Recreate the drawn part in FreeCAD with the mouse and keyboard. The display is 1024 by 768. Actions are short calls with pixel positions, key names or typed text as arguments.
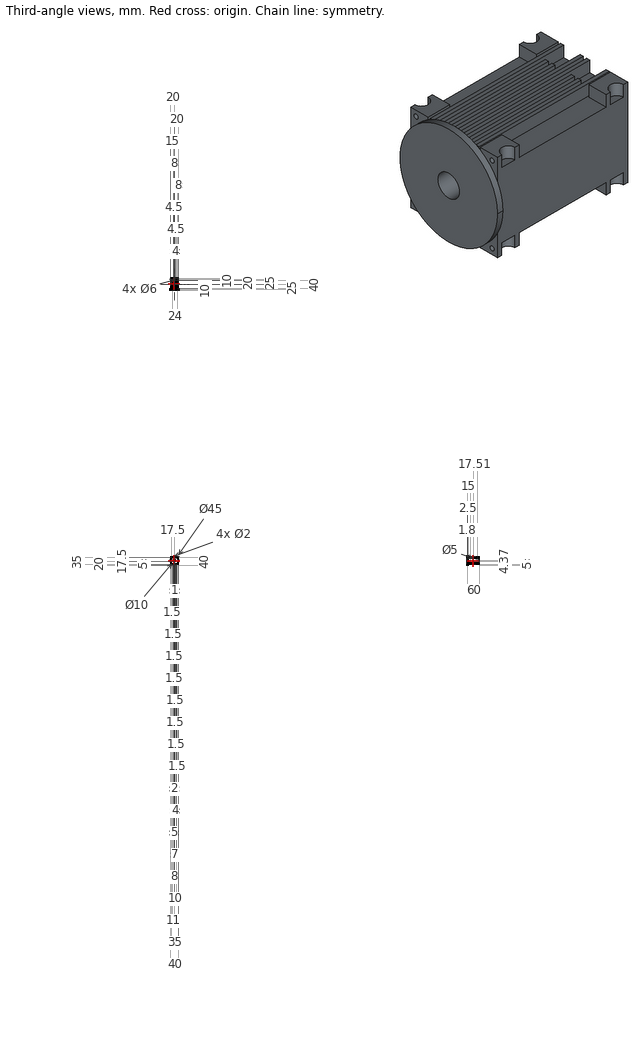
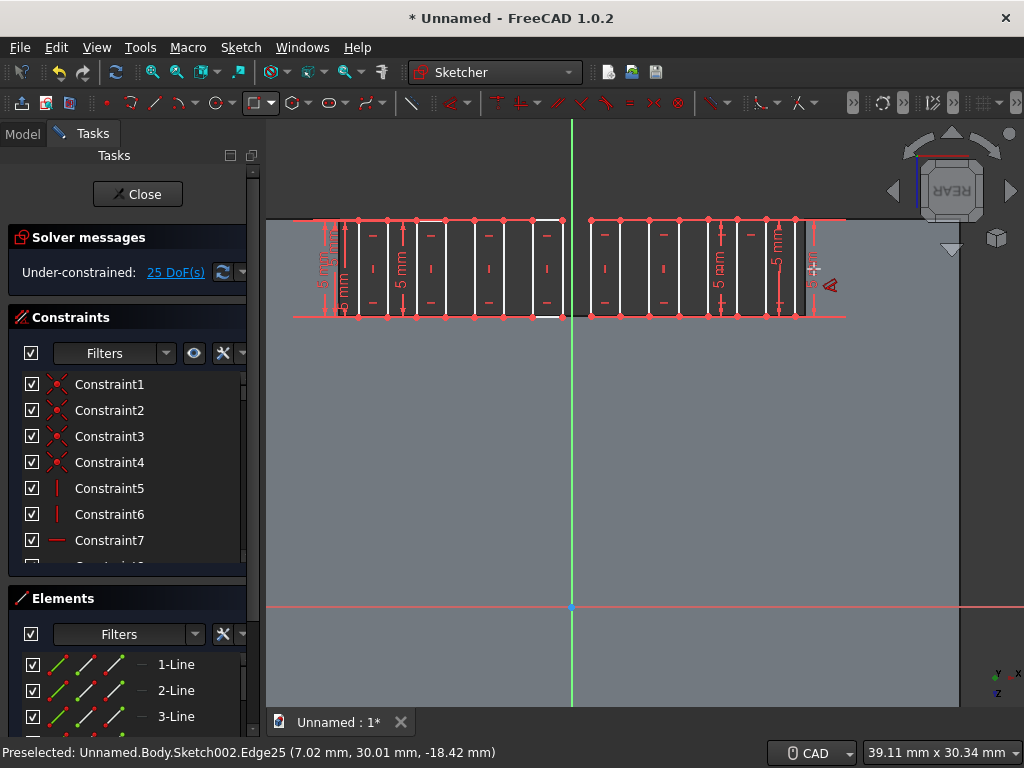
click(766, 249)
click(824, 291)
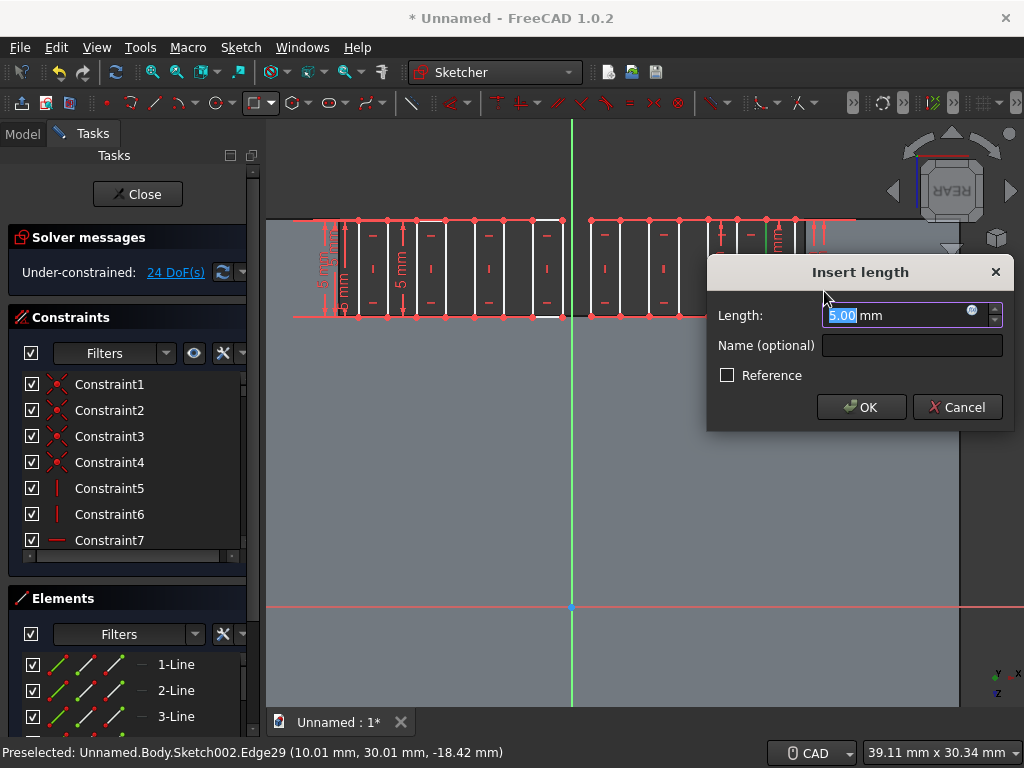
text(5)
key(Return)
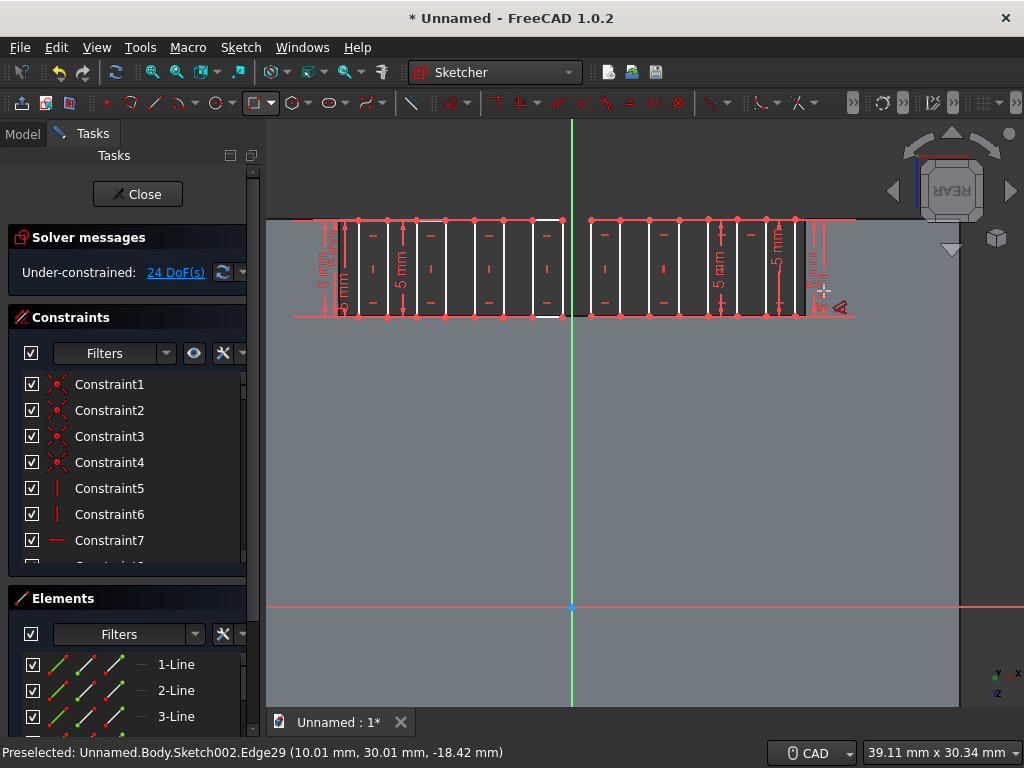
click(417, 221)
click(494, 641)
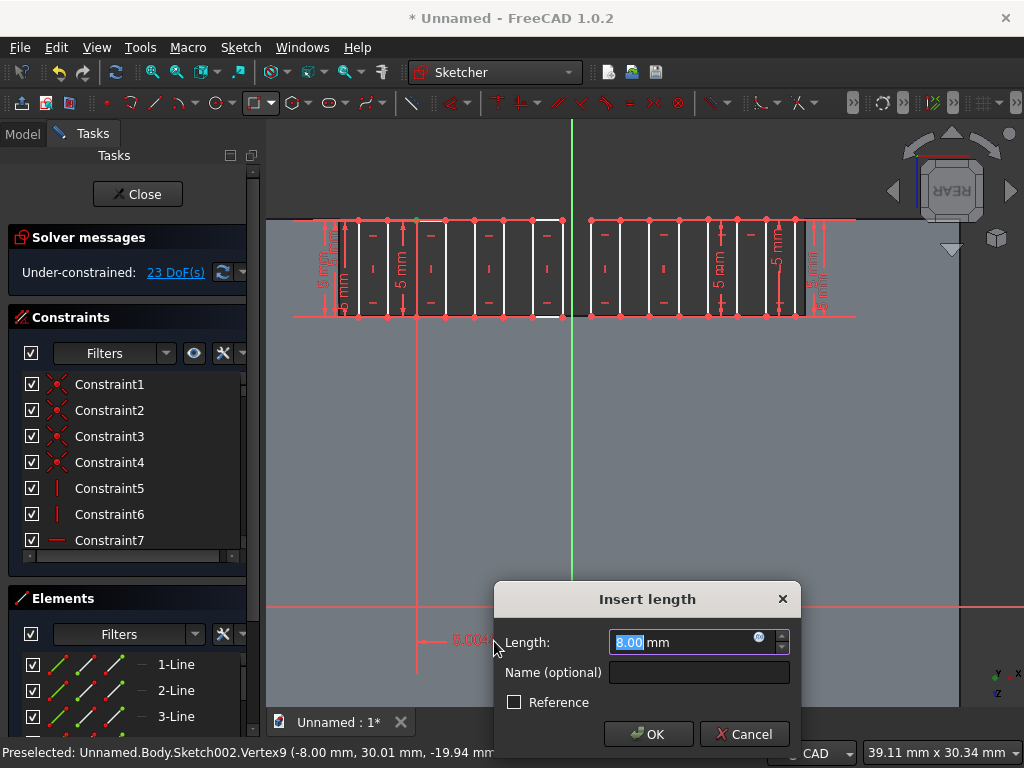
text(8)
key(Return)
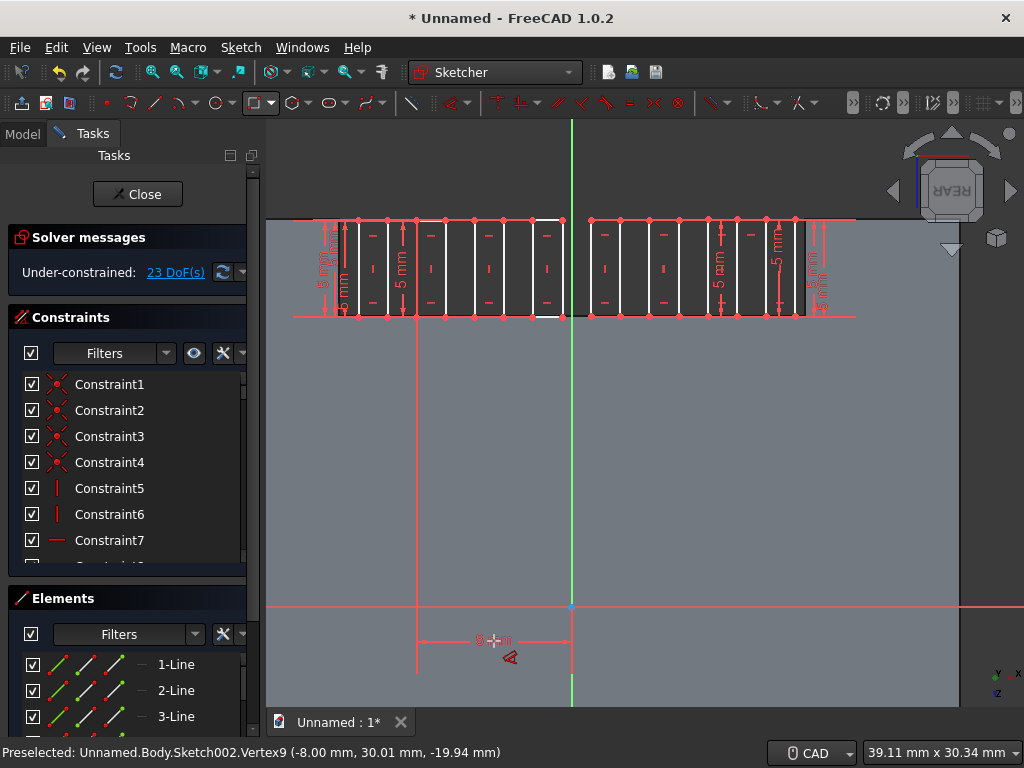
click(475, 220)
click(523, 186)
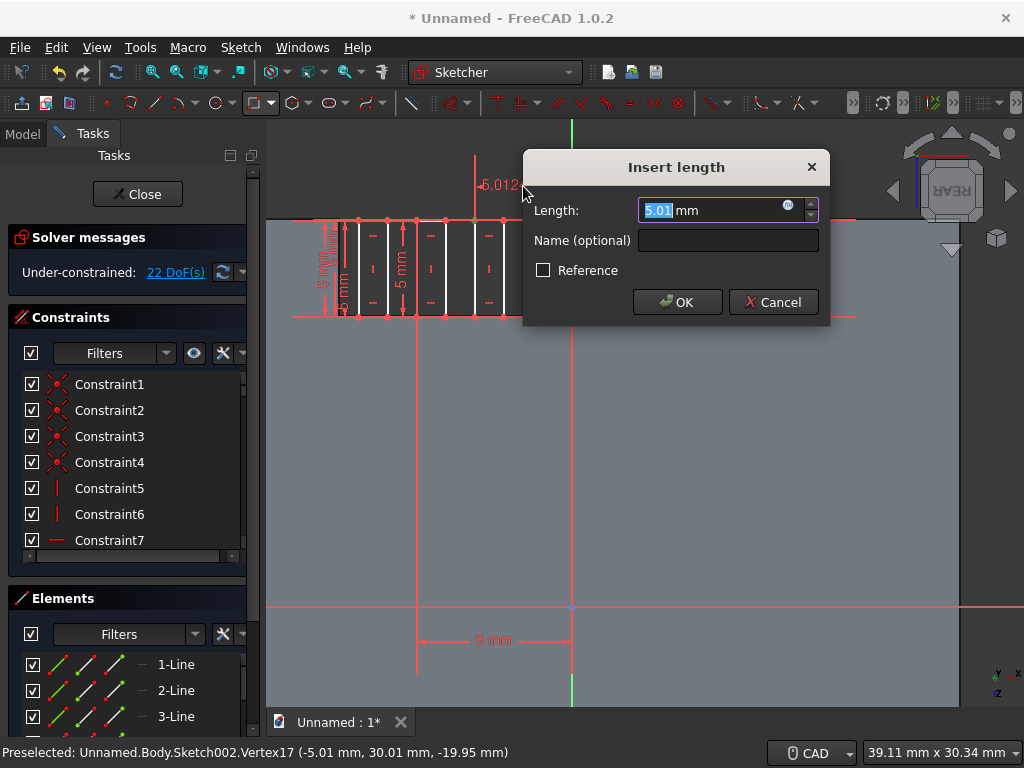
text(5)
key(Return)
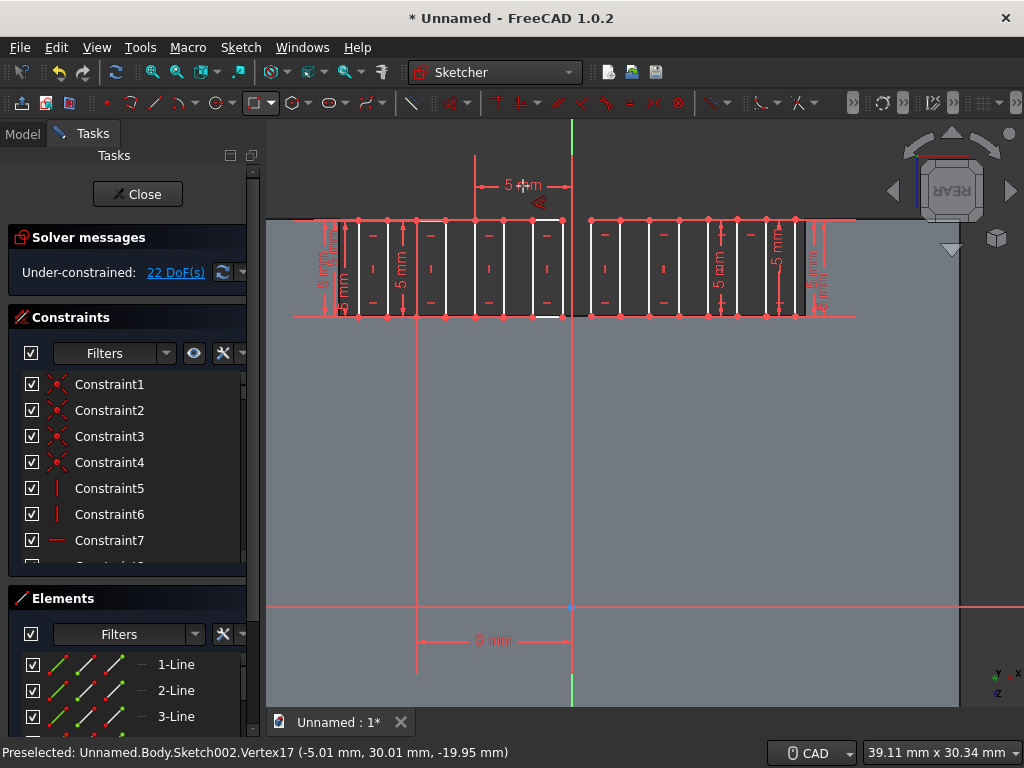
click(533, 220)
click(552, 665)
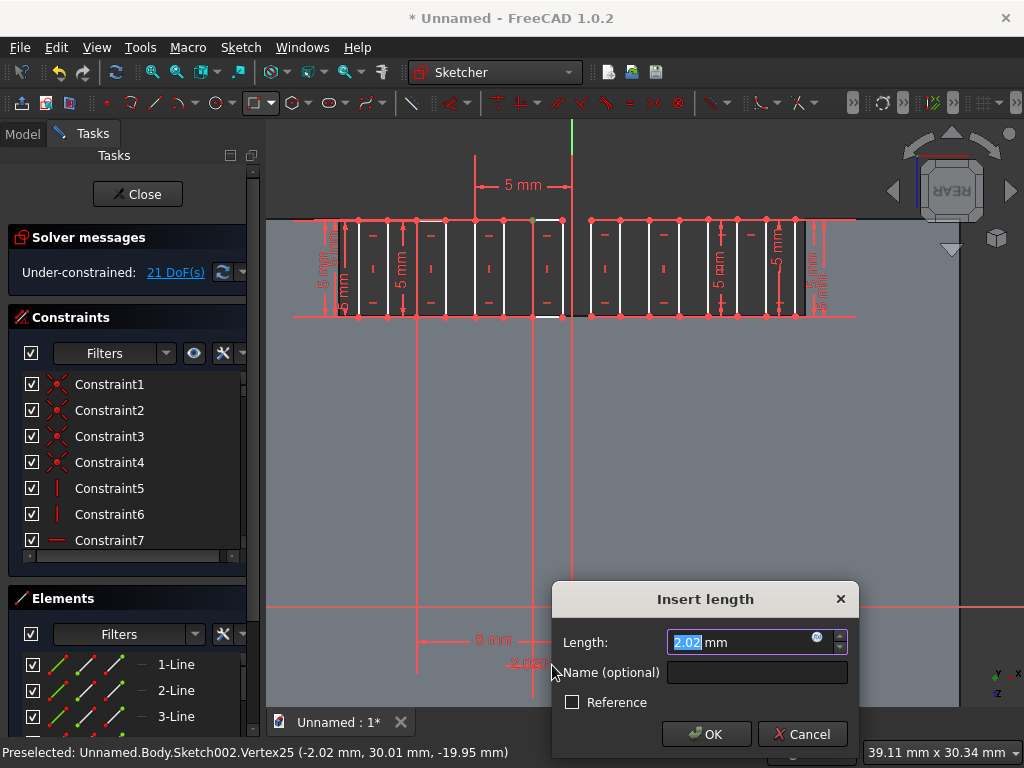
text(2)
key(Return)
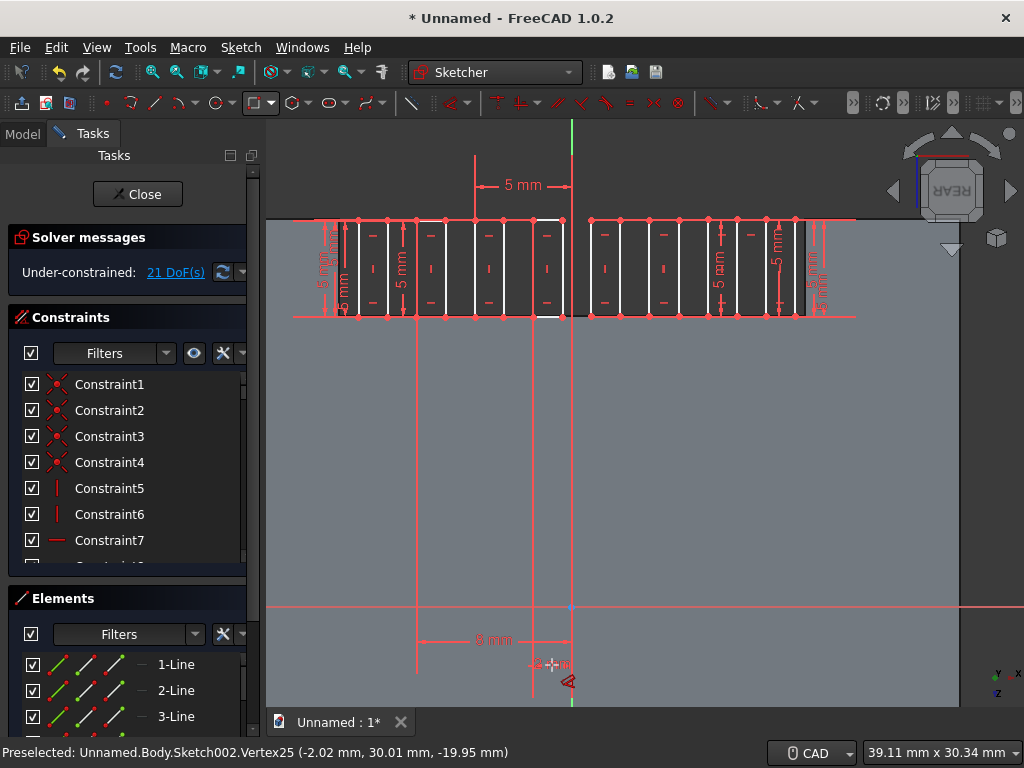
scroll(591, 220, up, 4)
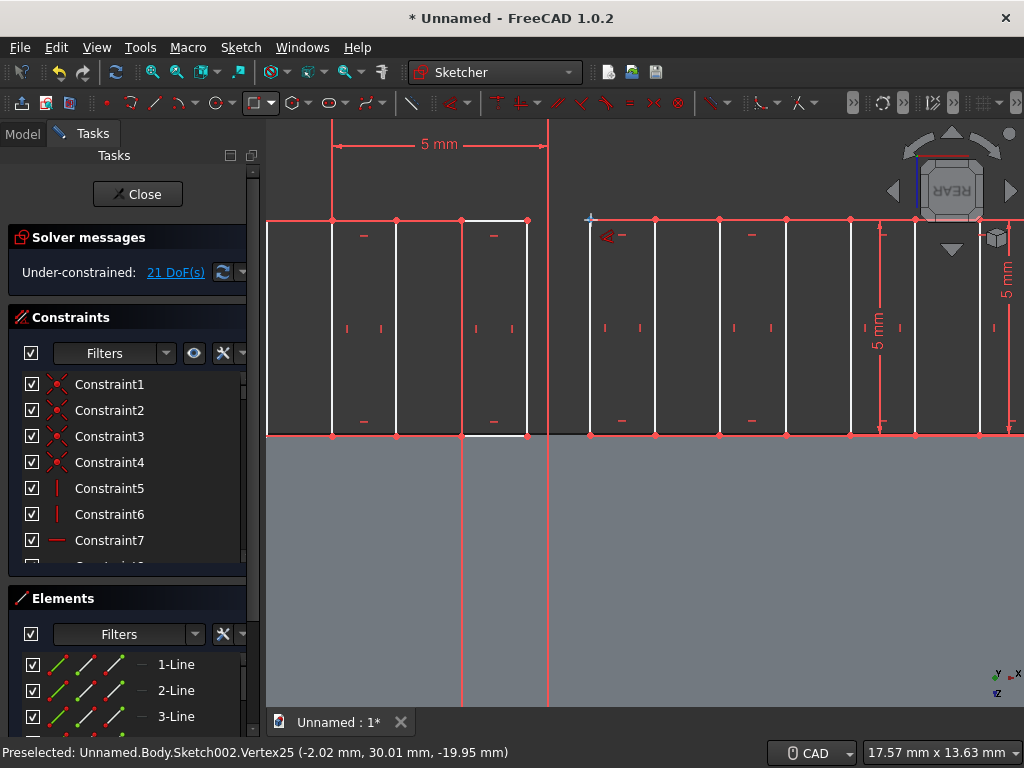
click(590, 220)
click(569, 186)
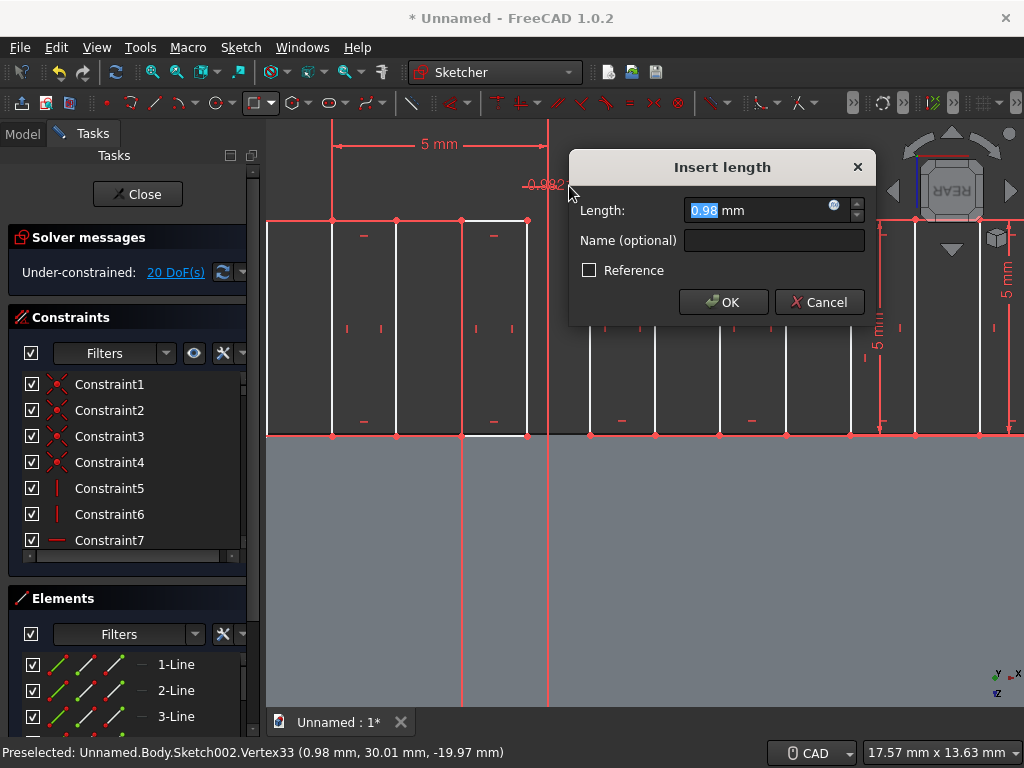
text(1)
key(Return)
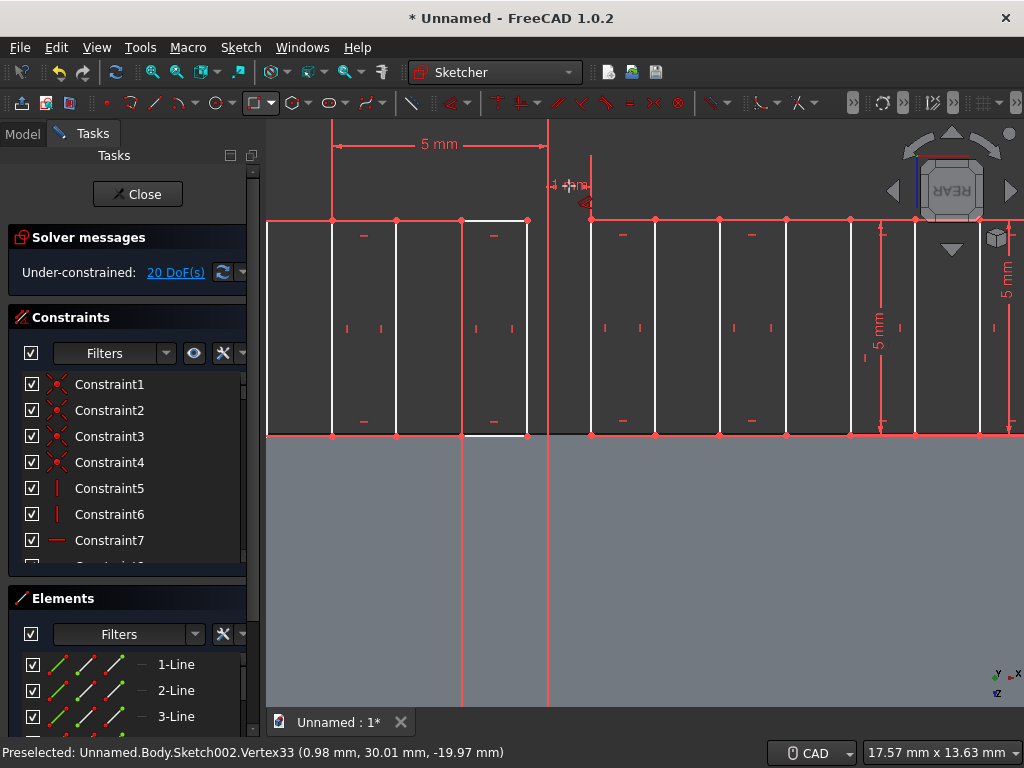
click(720, 220)
click(673, 186)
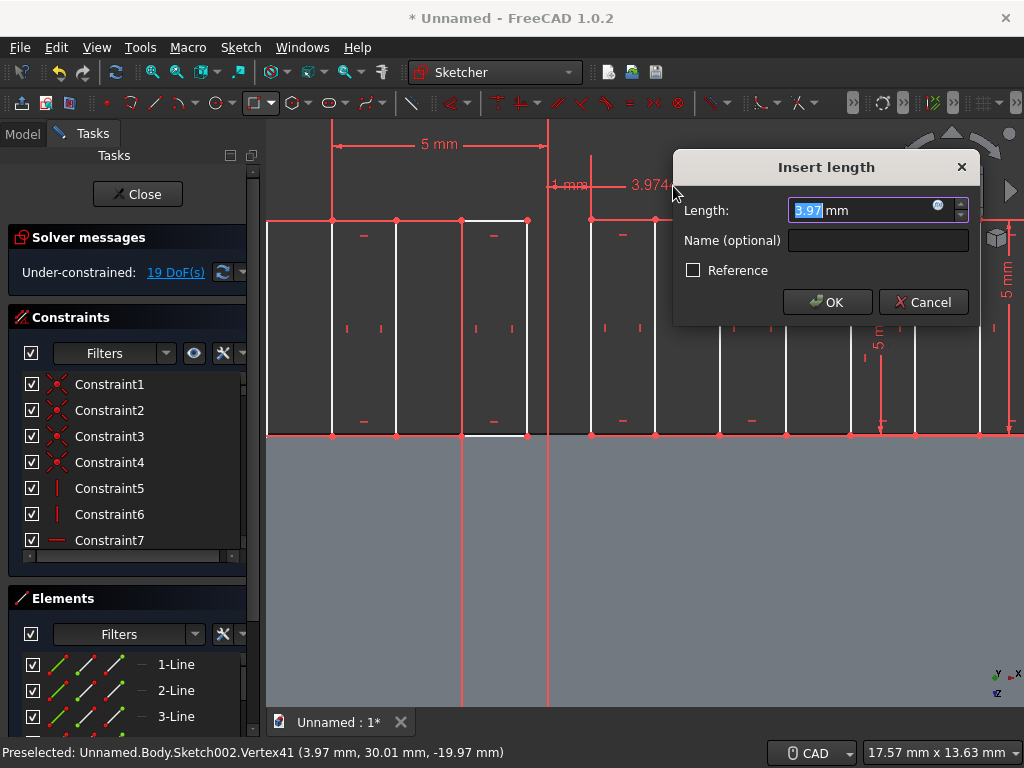
text(4)
key(Return)